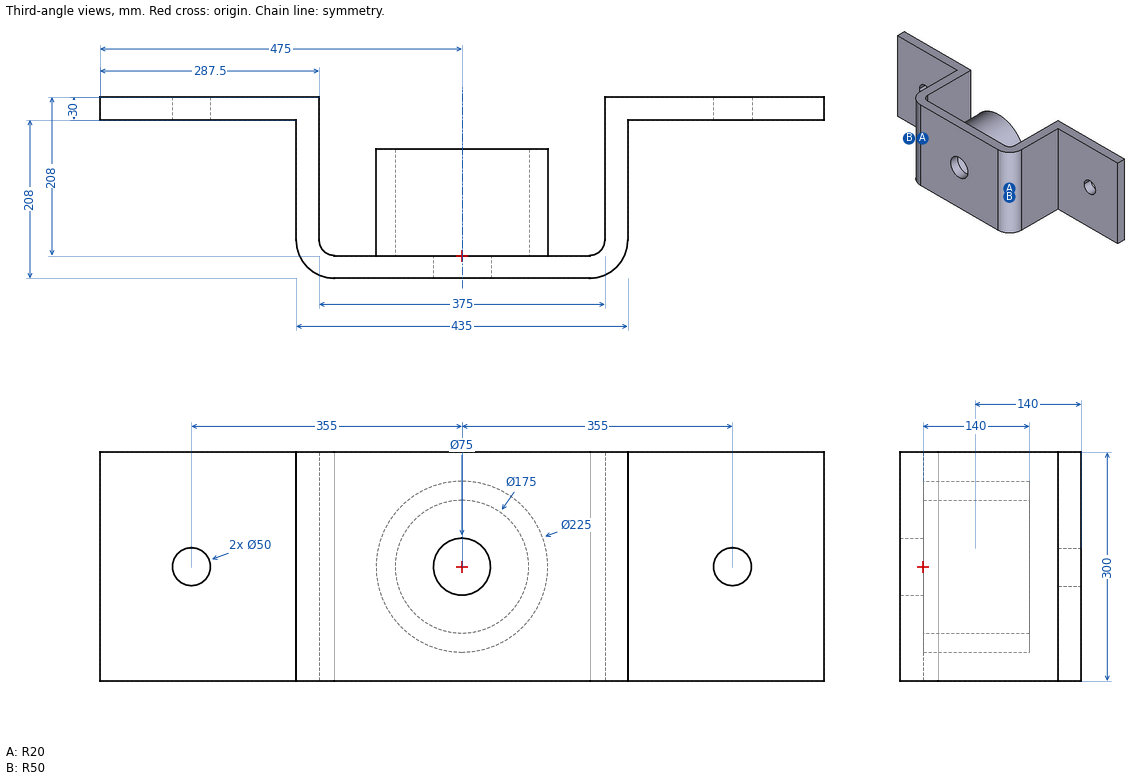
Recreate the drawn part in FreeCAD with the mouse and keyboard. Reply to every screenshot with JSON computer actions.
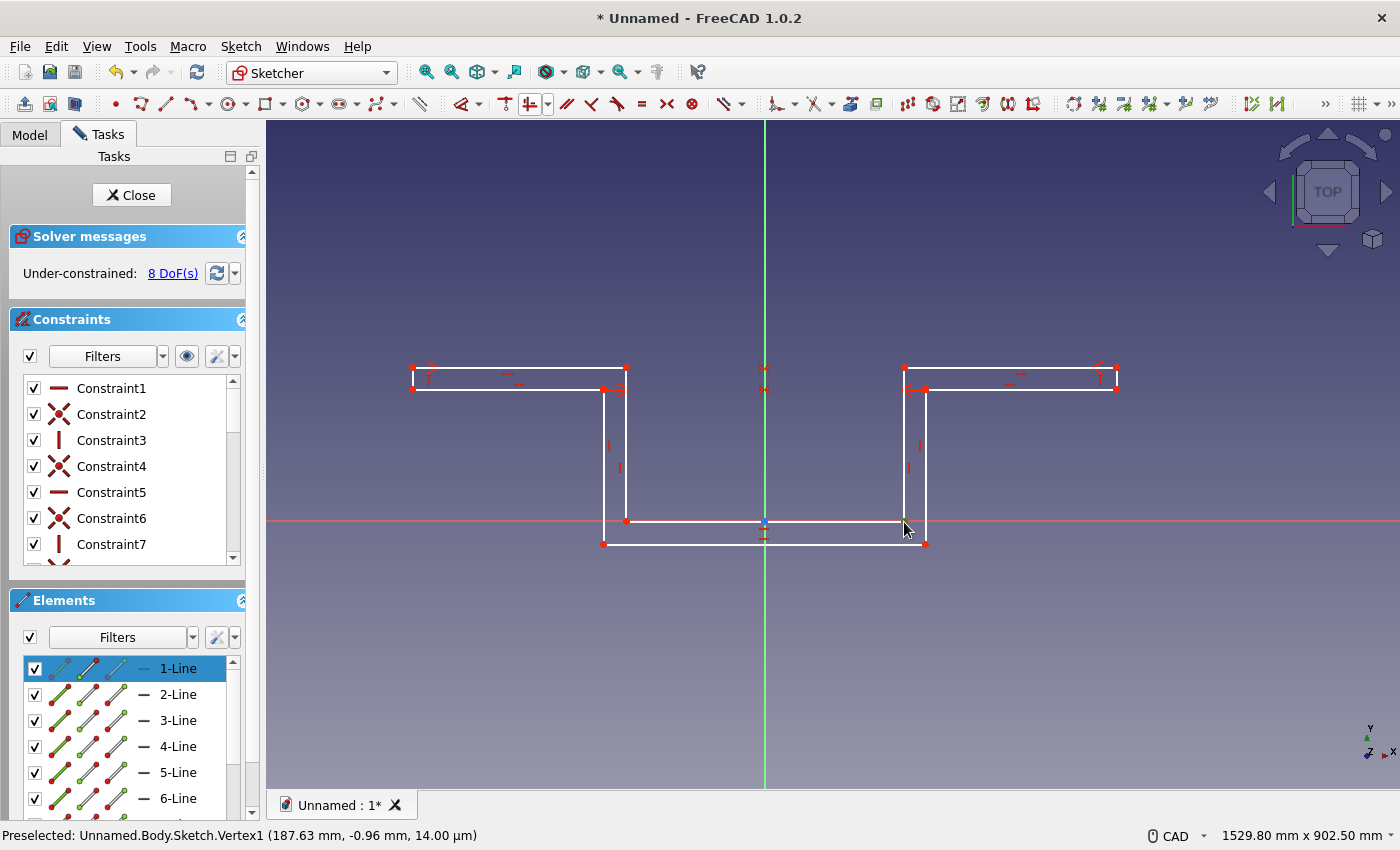
{"action": "left_click", "coordinate": [361, 521]}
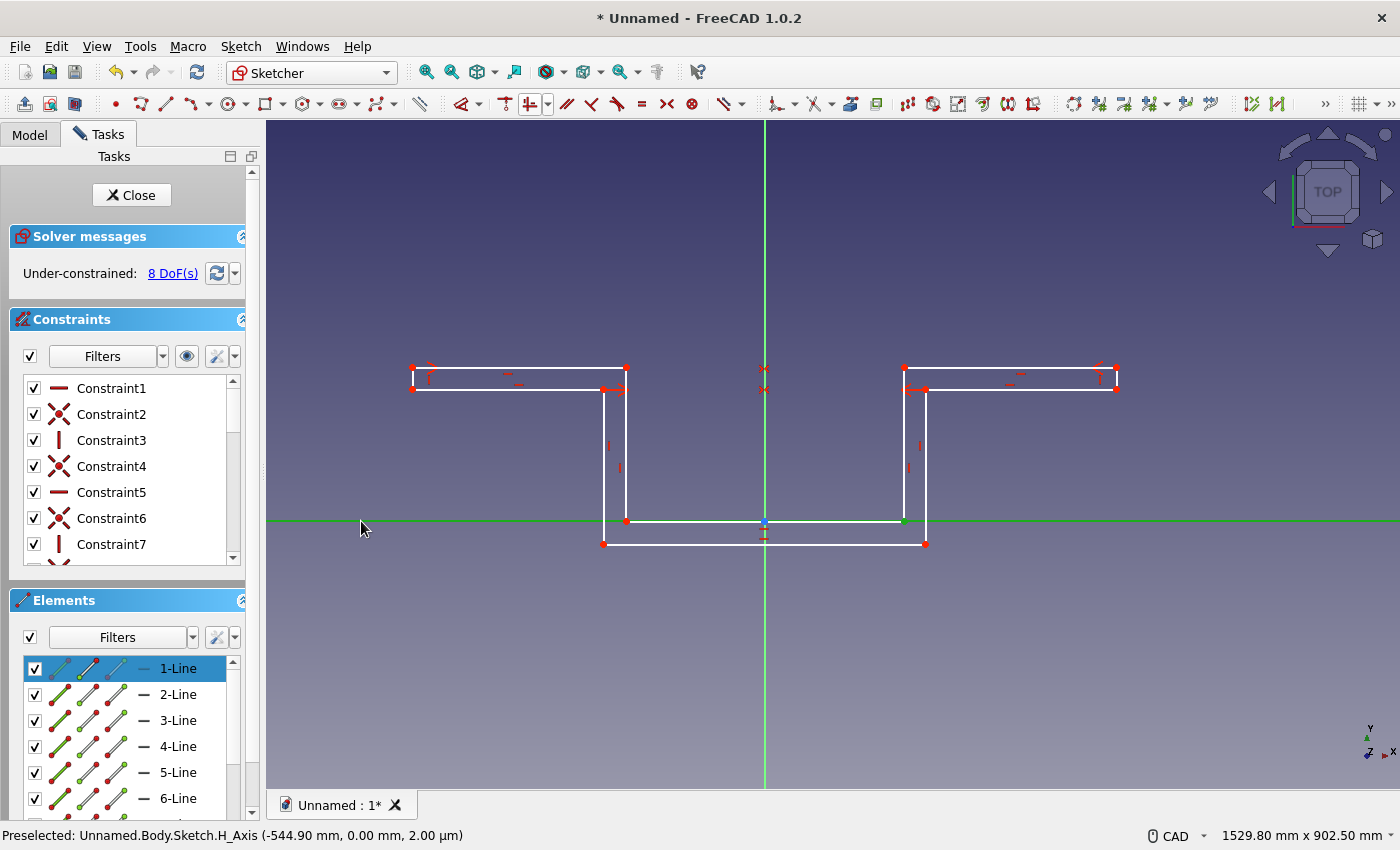
{"action": "left_click", "coordinate": [505, 104]}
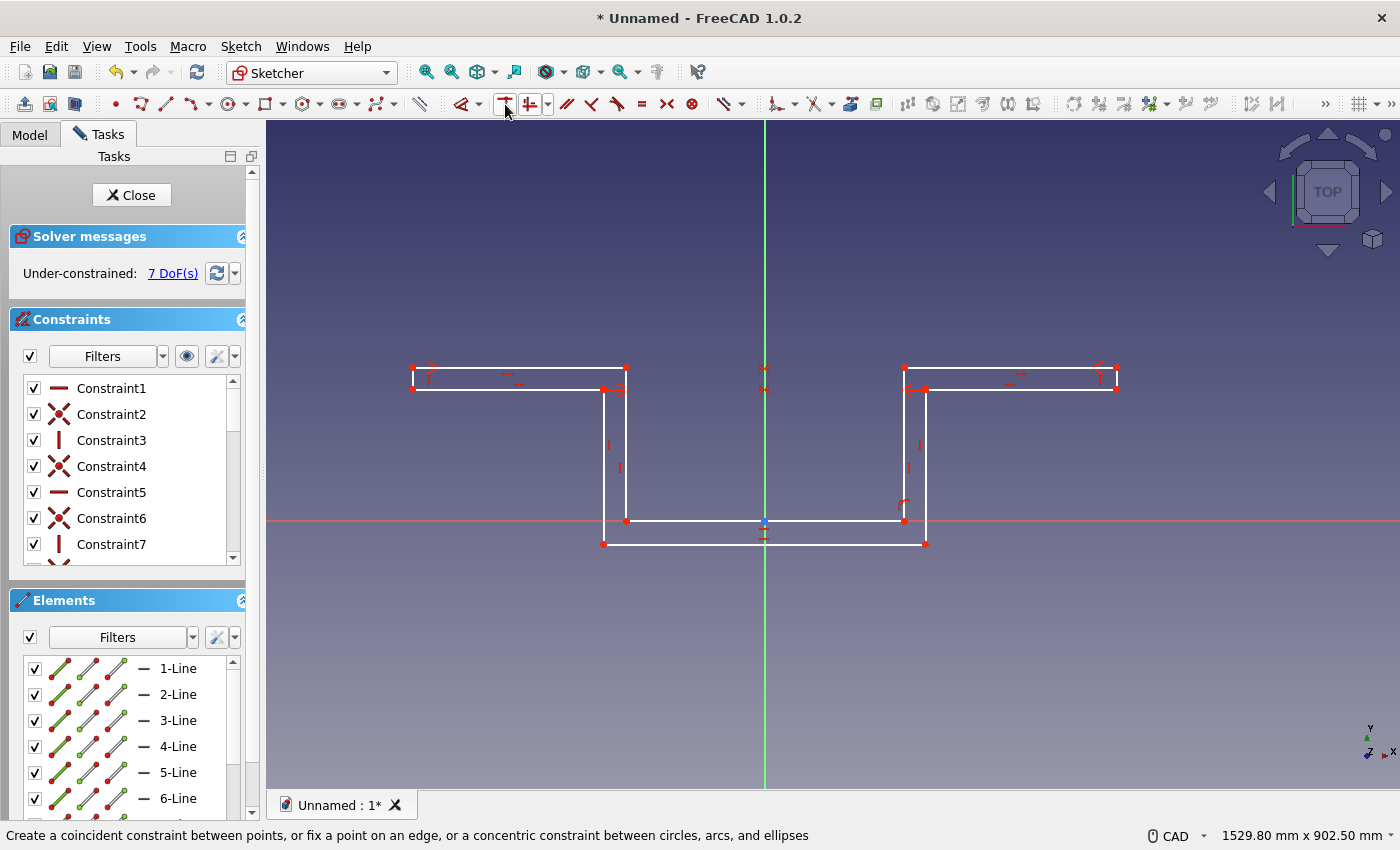
{"action": "scroll", "coordinate": [413, 379], "scroll_direction": "up", "scroll_amount": 3}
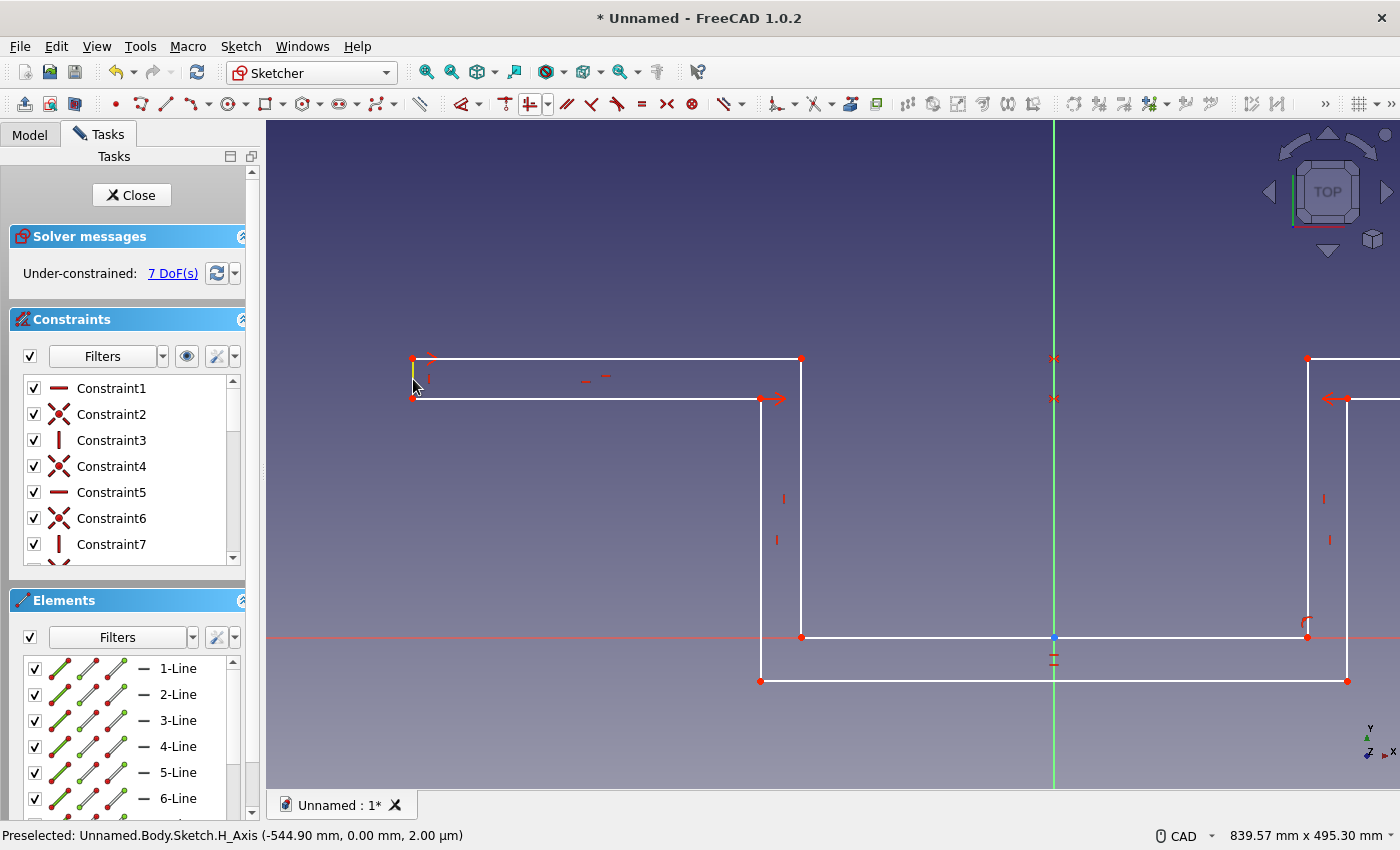
{"action": "left_click", "coordinate": [413, 379]}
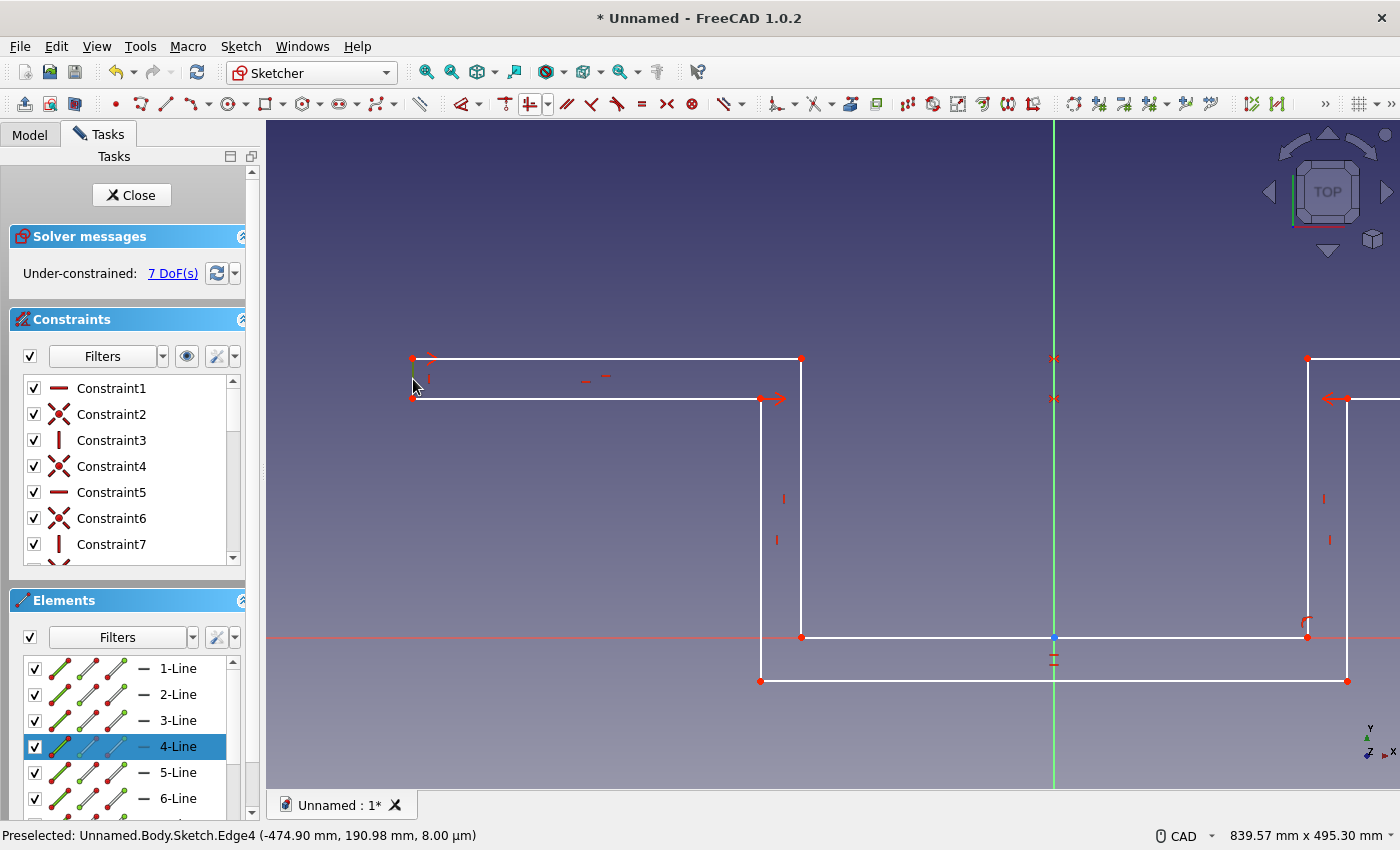
{"action": "left_click", "coordinate": [478, 104]}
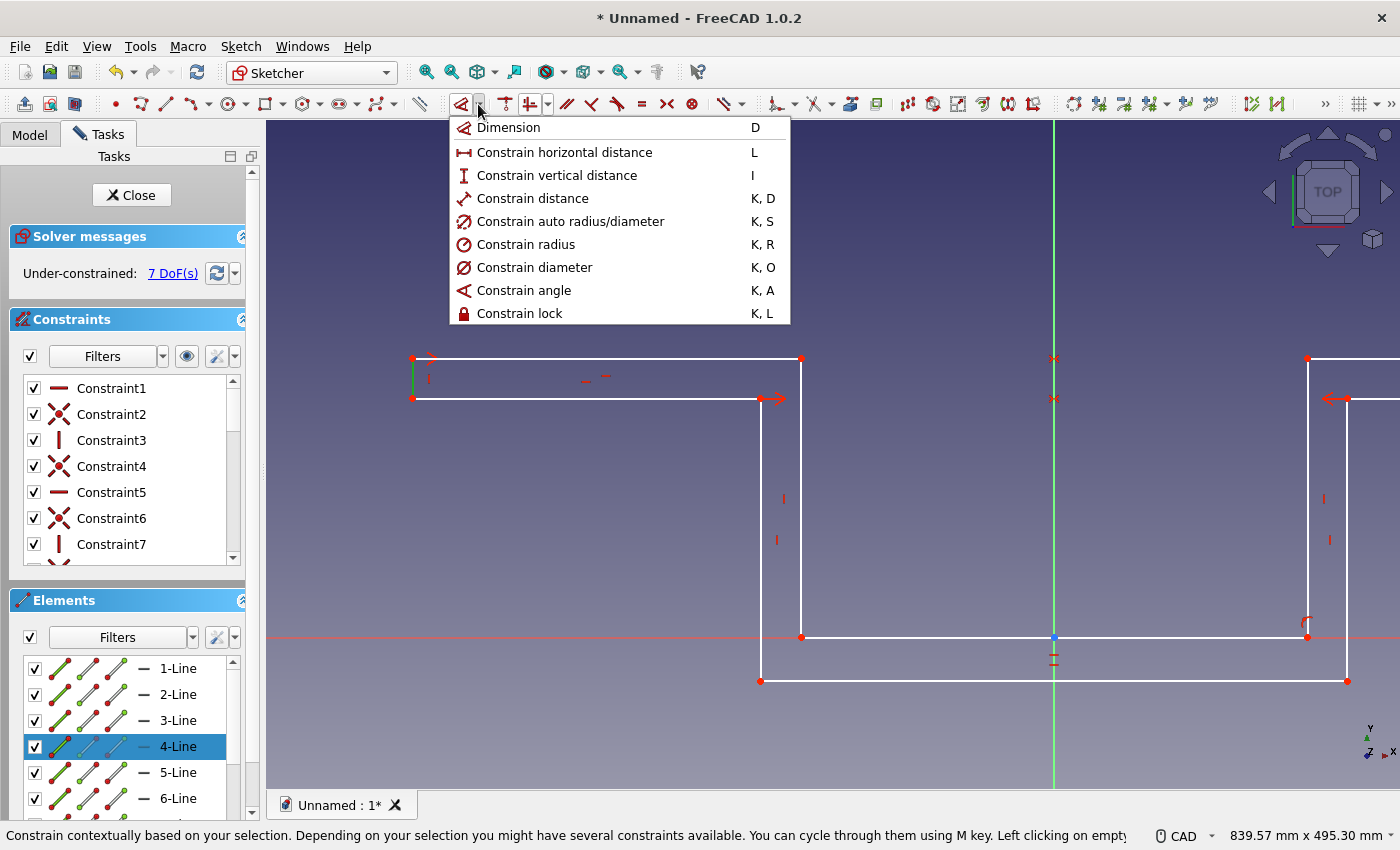
{"action": "left_click", "coordinate": [620, 176]}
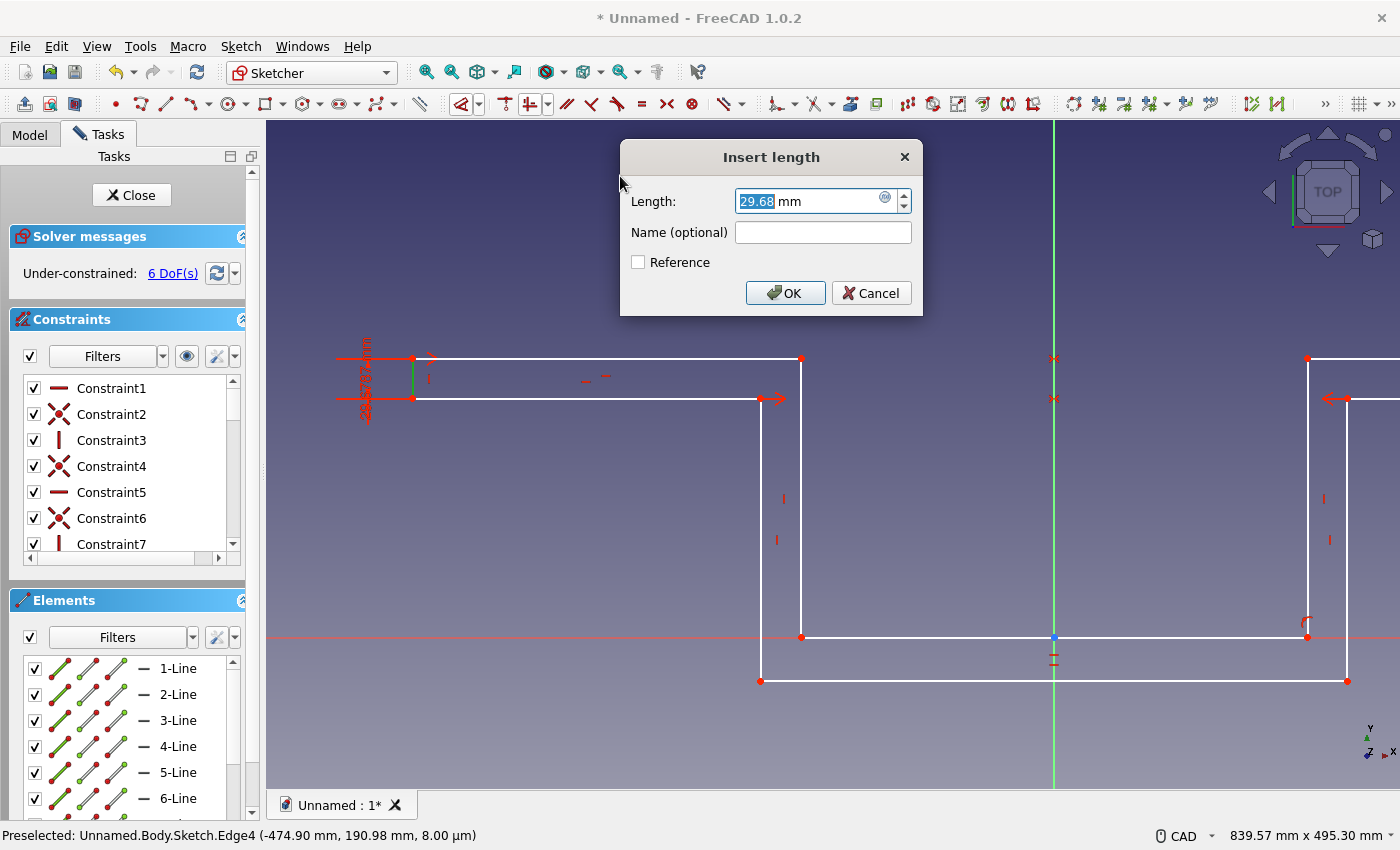
{"action": "type", "text": "30"}
{"action": "key", "text": "Return"}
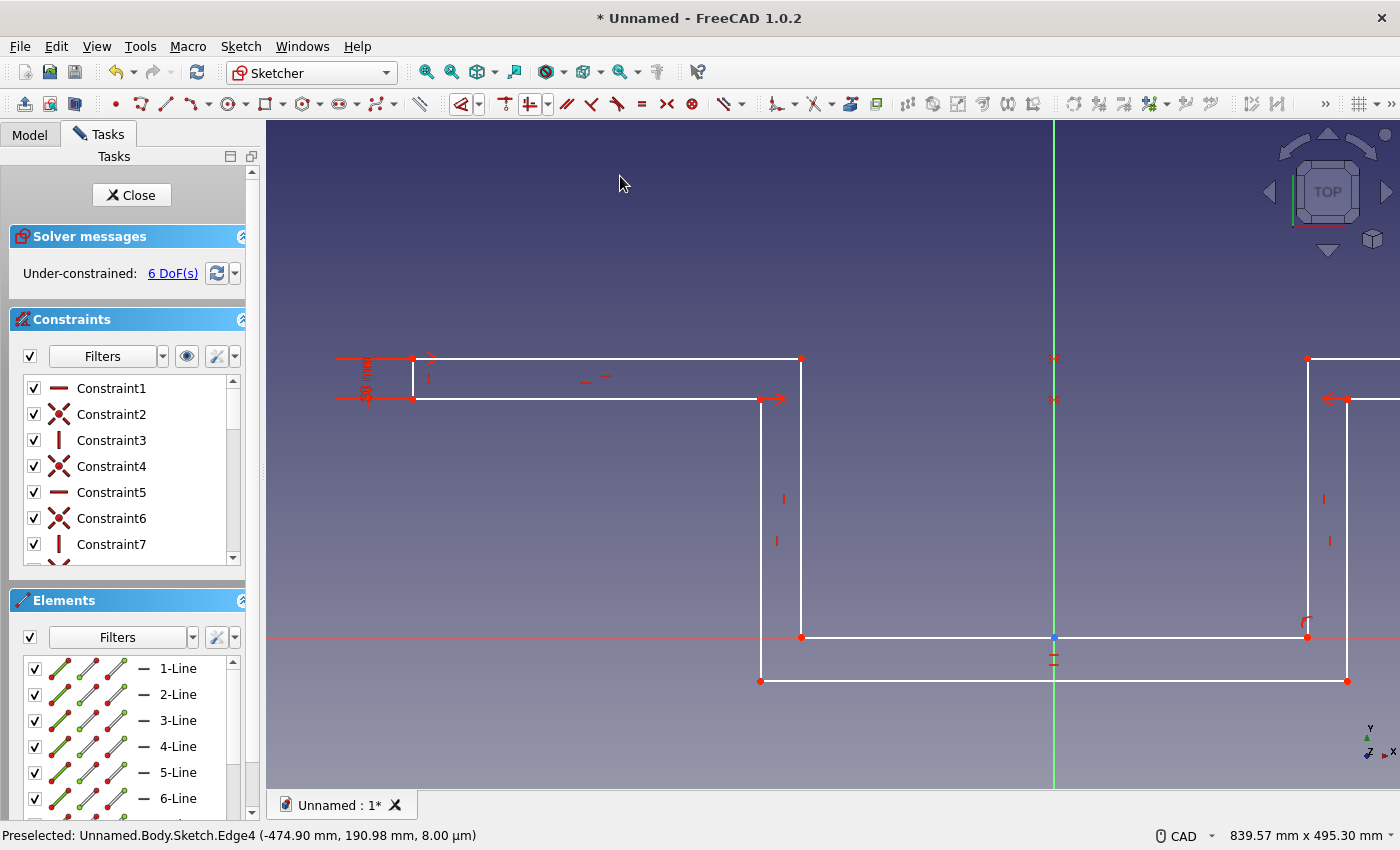
{"action": "left_click", "coordinate": [1156, 638]}